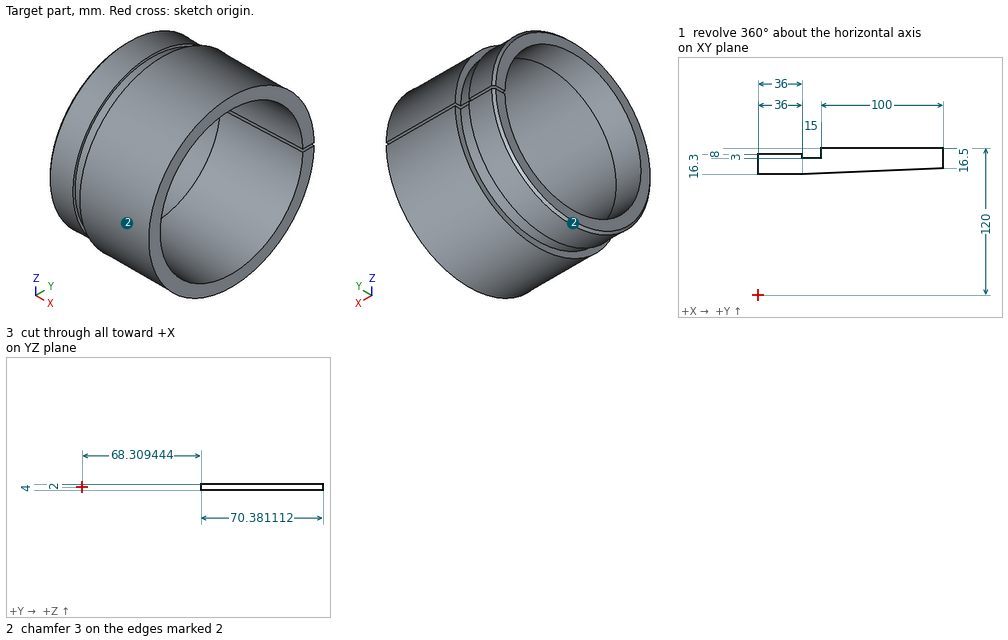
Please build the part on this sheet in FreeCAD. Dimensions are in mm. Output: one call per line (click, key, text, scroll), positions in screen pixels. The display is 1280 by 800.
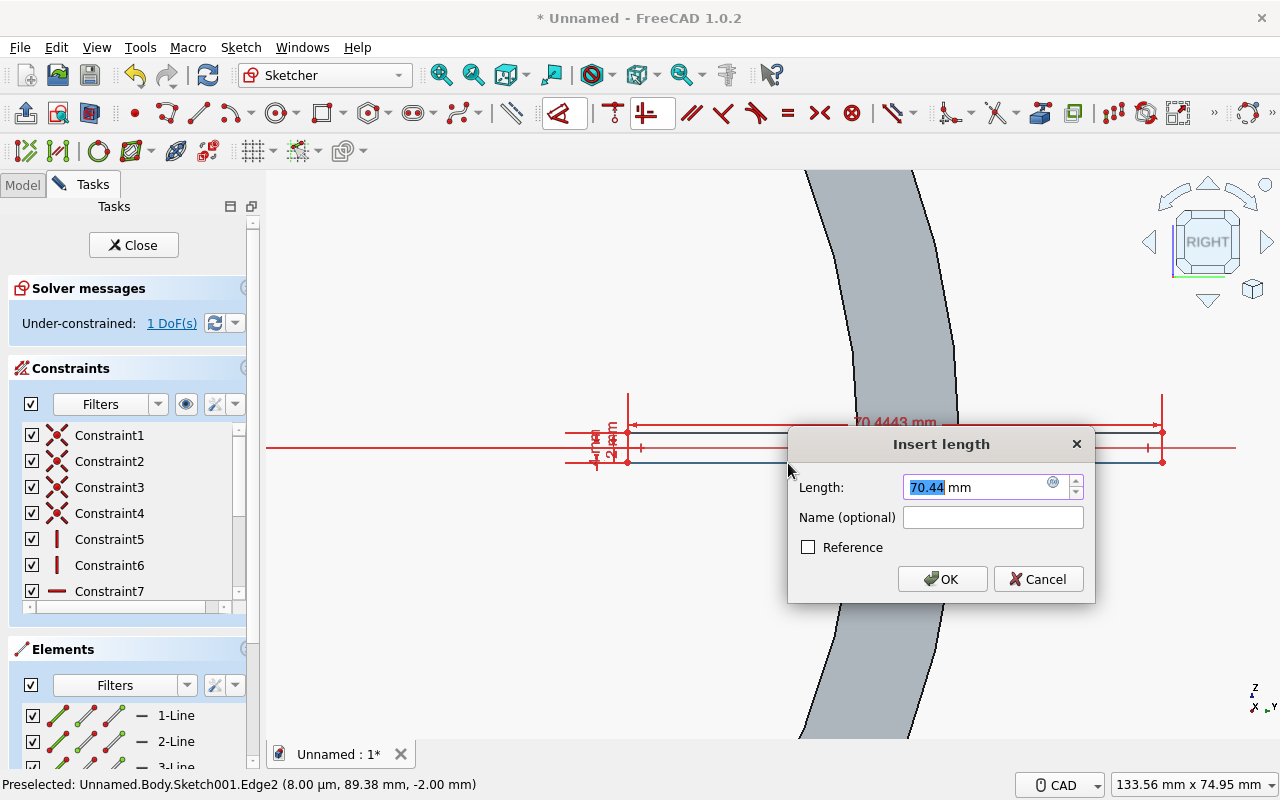
text(70.381112)
key(Return)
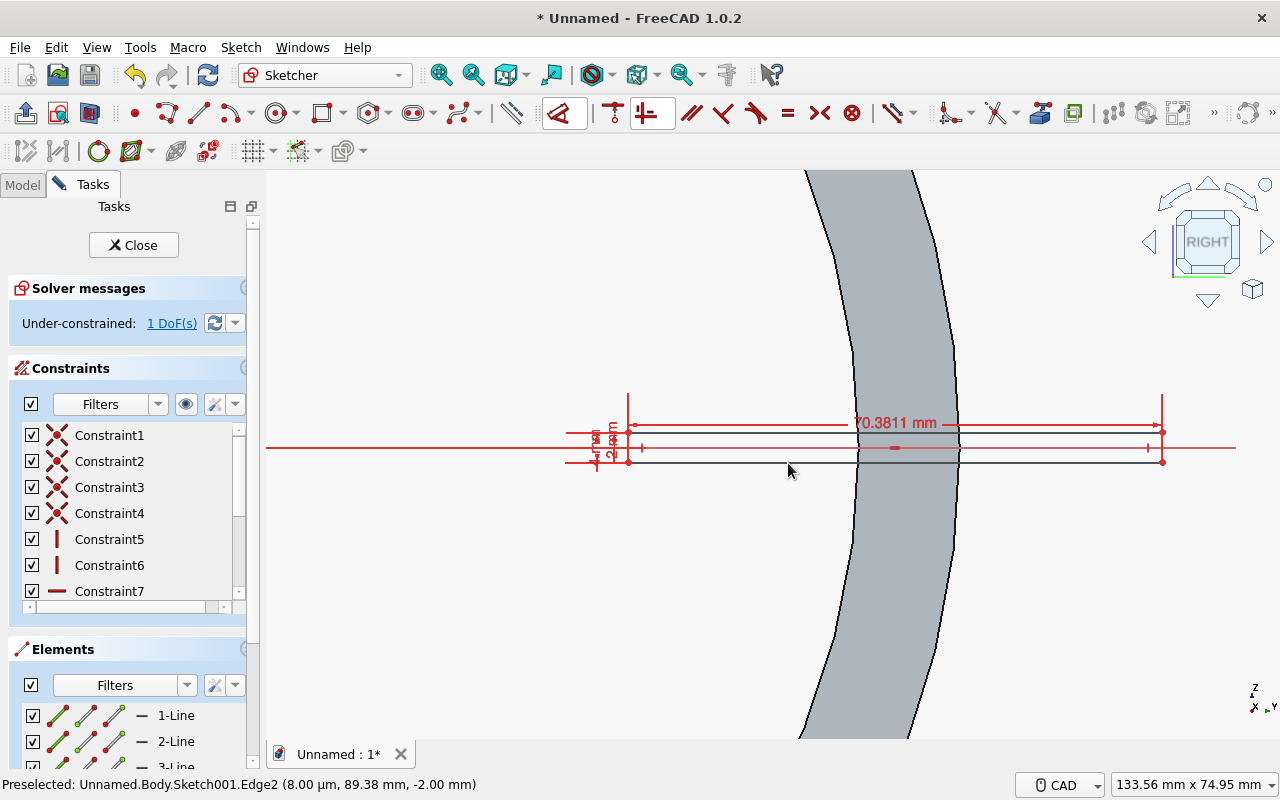
click(628, 433)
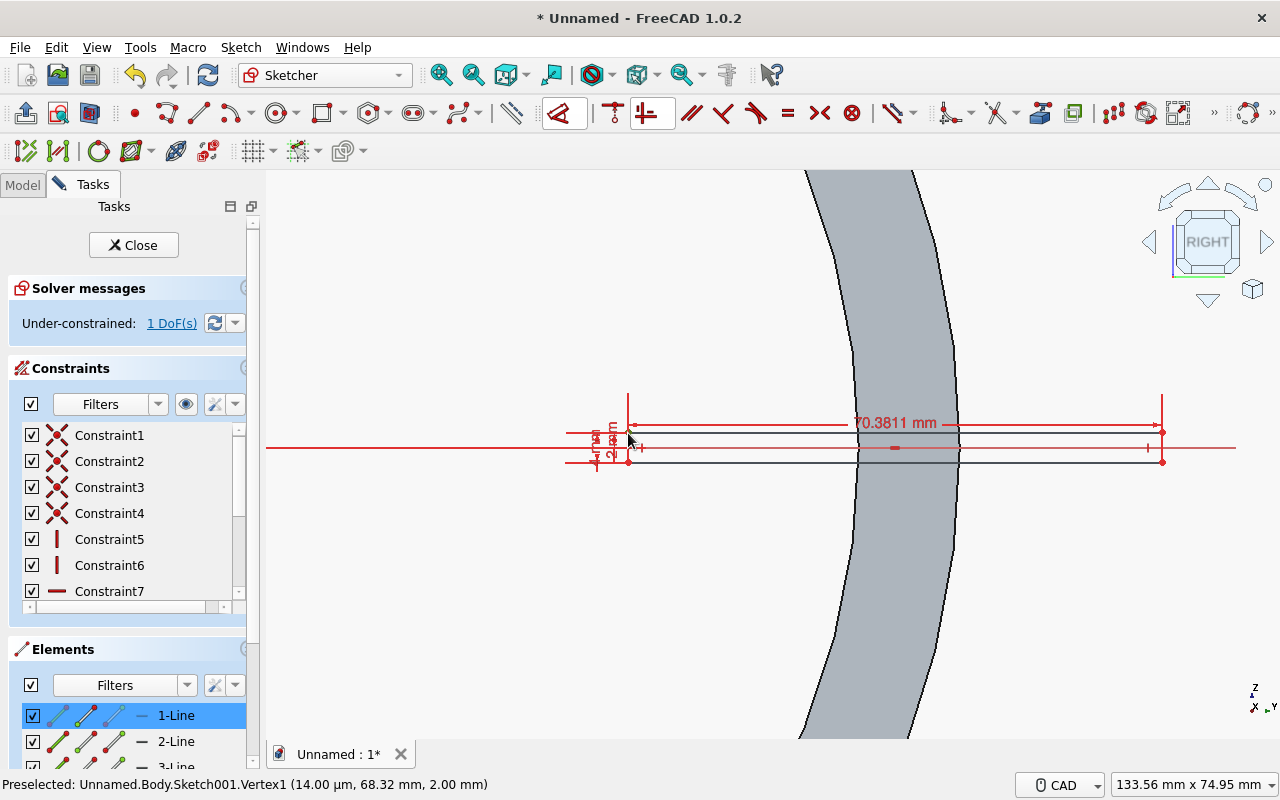
click(582, 114)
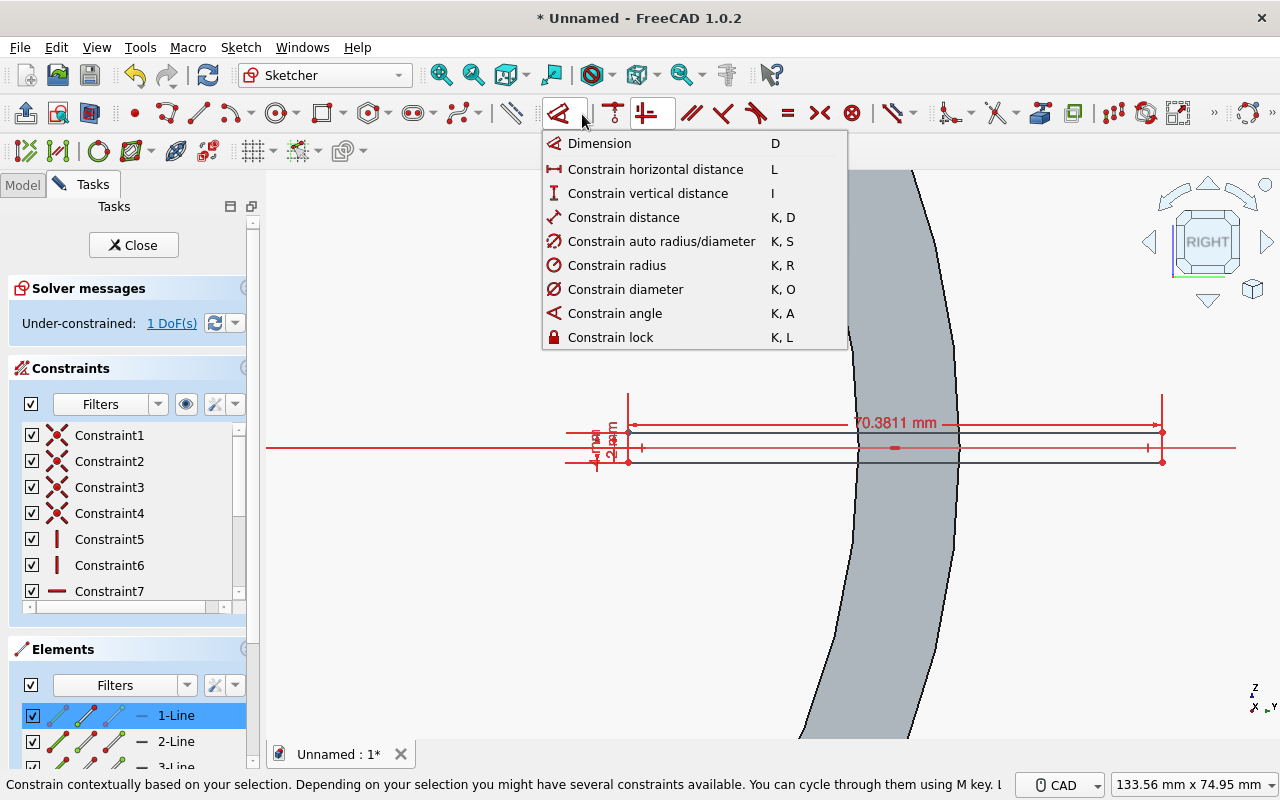
click(695, 169)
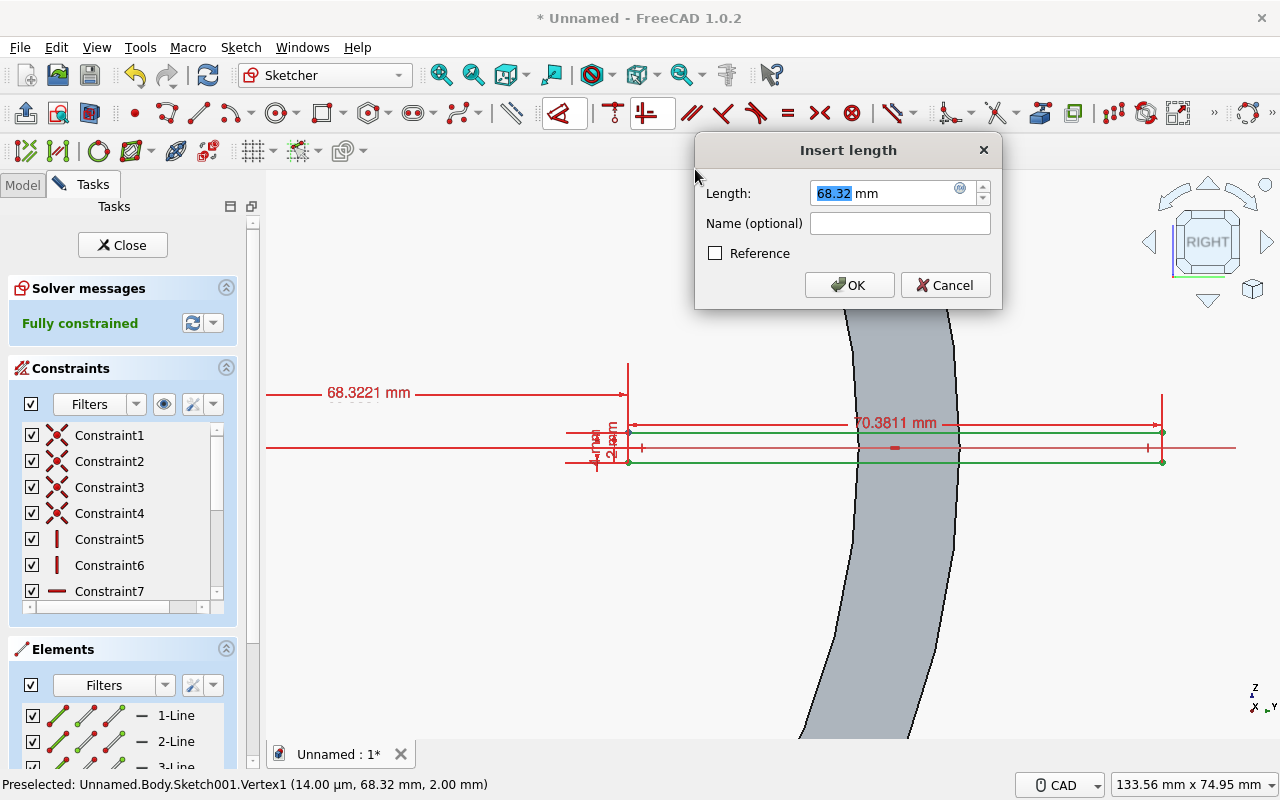
text(68.309444)
key(Return)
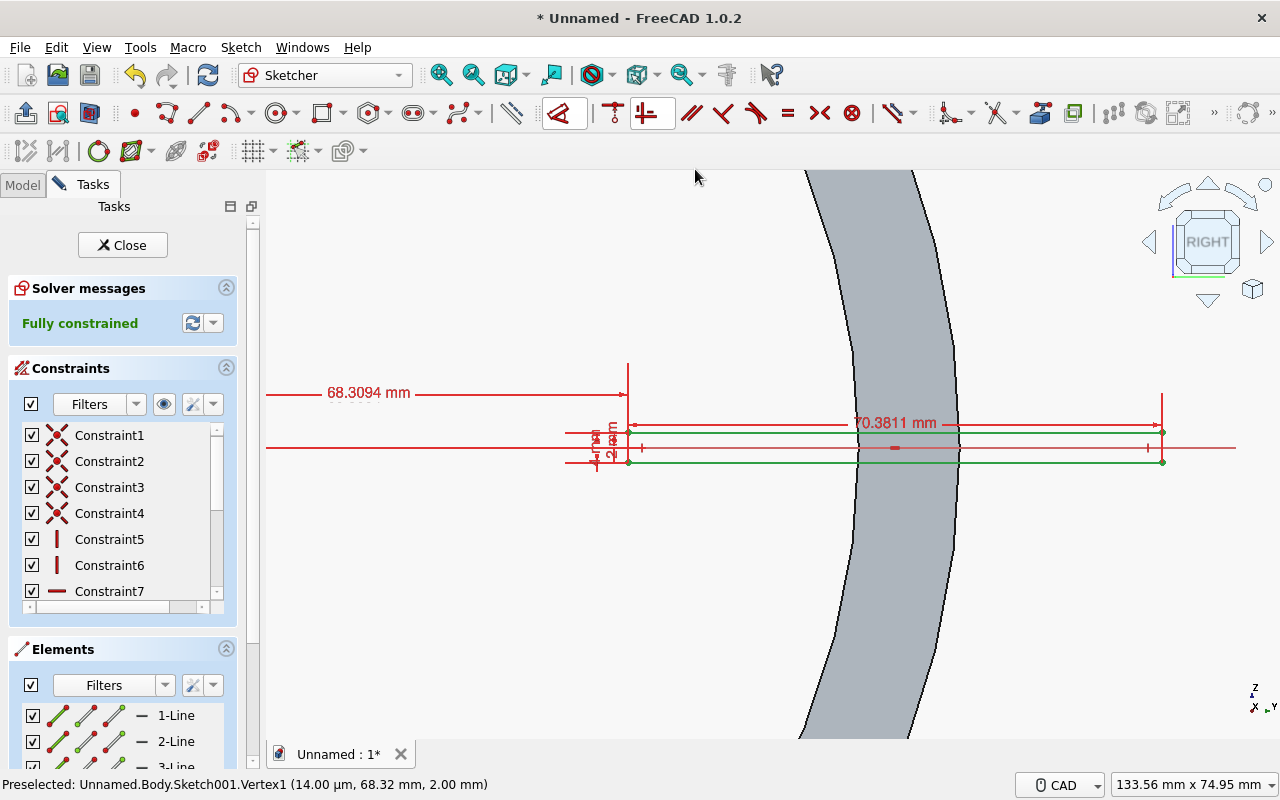
click(123, 245)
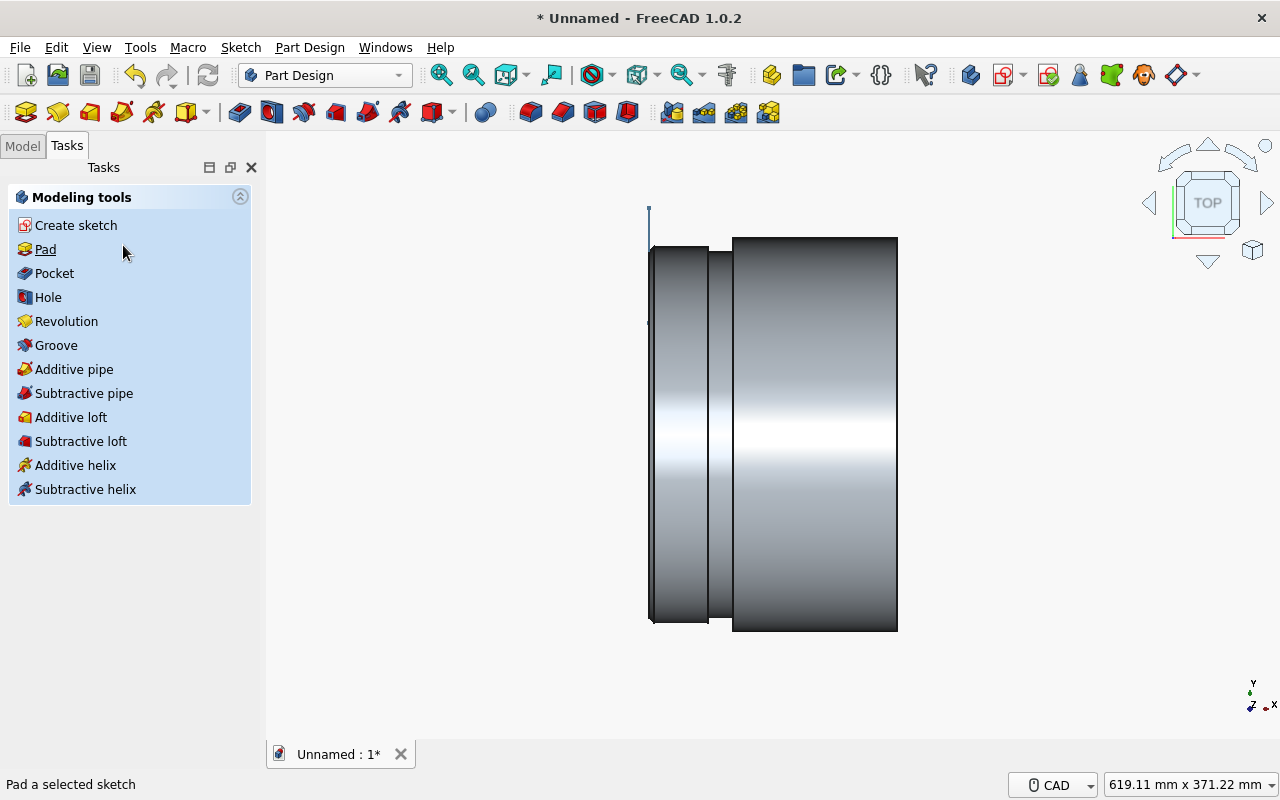
click(240, 112)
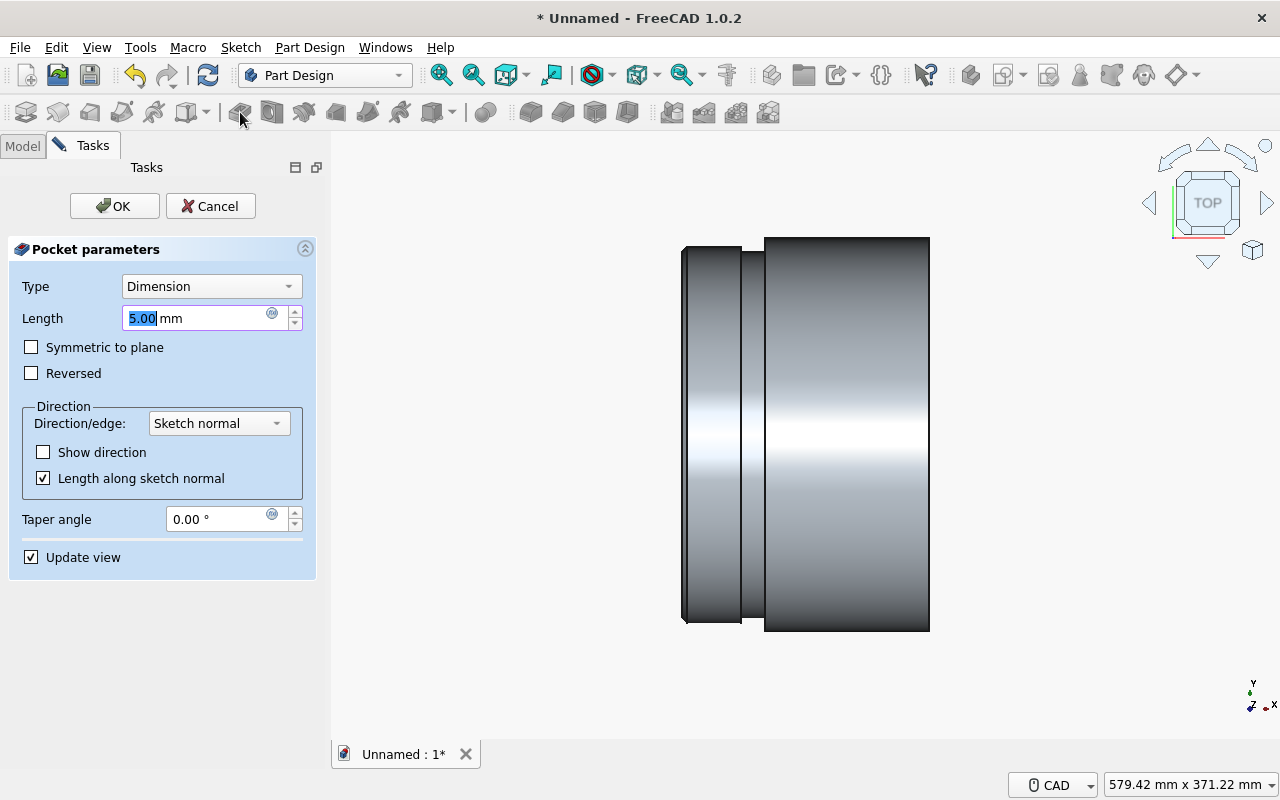
click(212, 286)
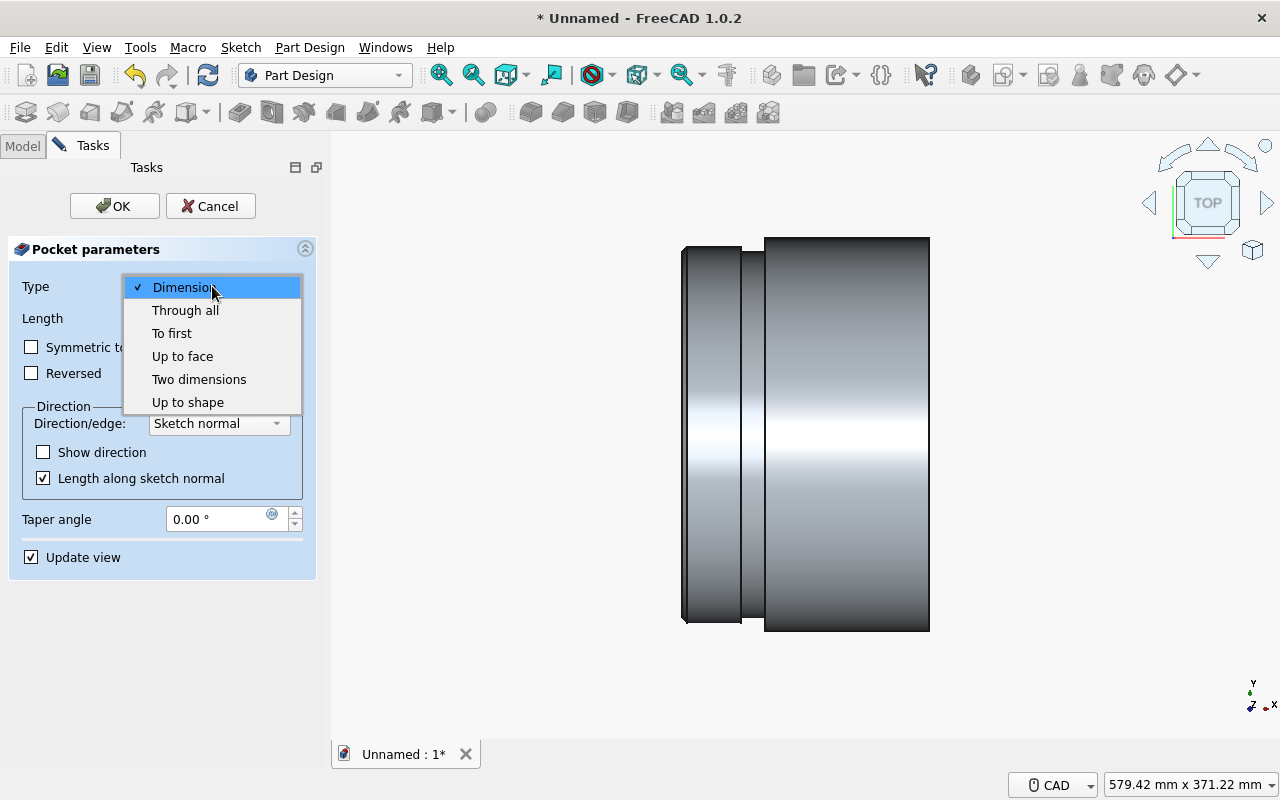
click(212, 310)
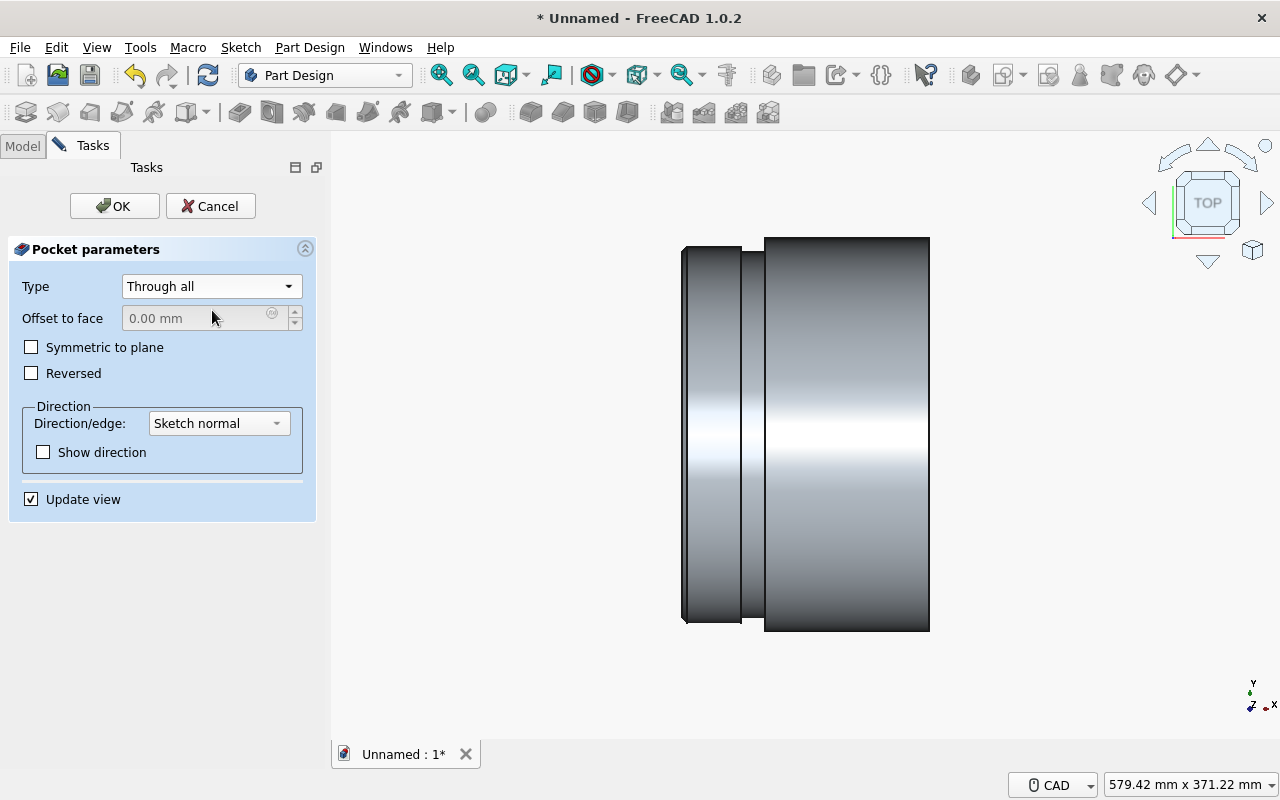
click(30, 373)